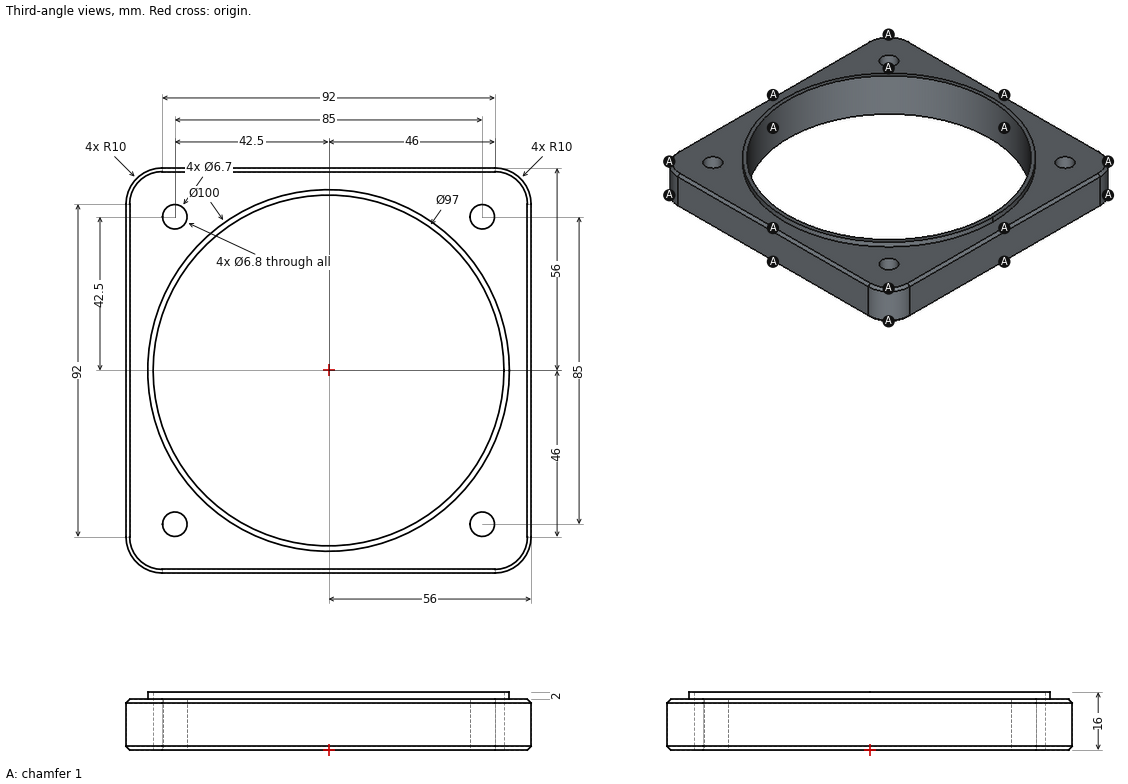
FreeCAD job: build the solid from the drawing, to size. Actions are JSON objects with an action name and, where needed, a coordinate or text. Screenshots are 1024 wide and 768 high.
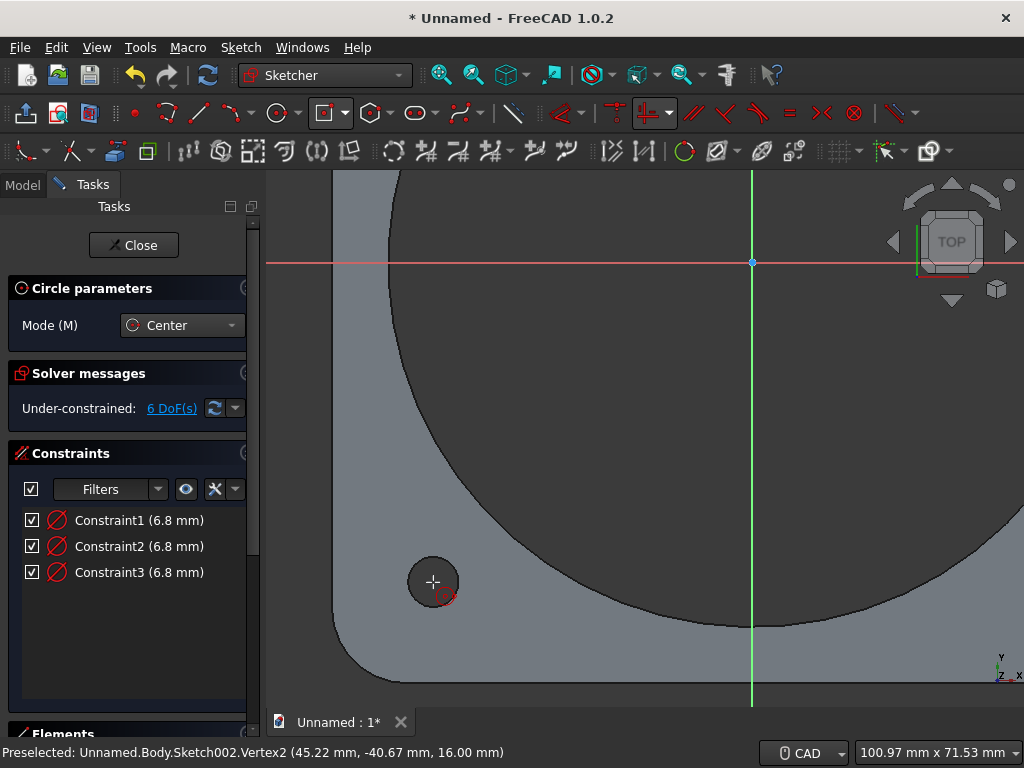
{"action": "left_click", "coordinate": [433, 582]}
{"action": "mouse_move", "coordinate": [451, 564]}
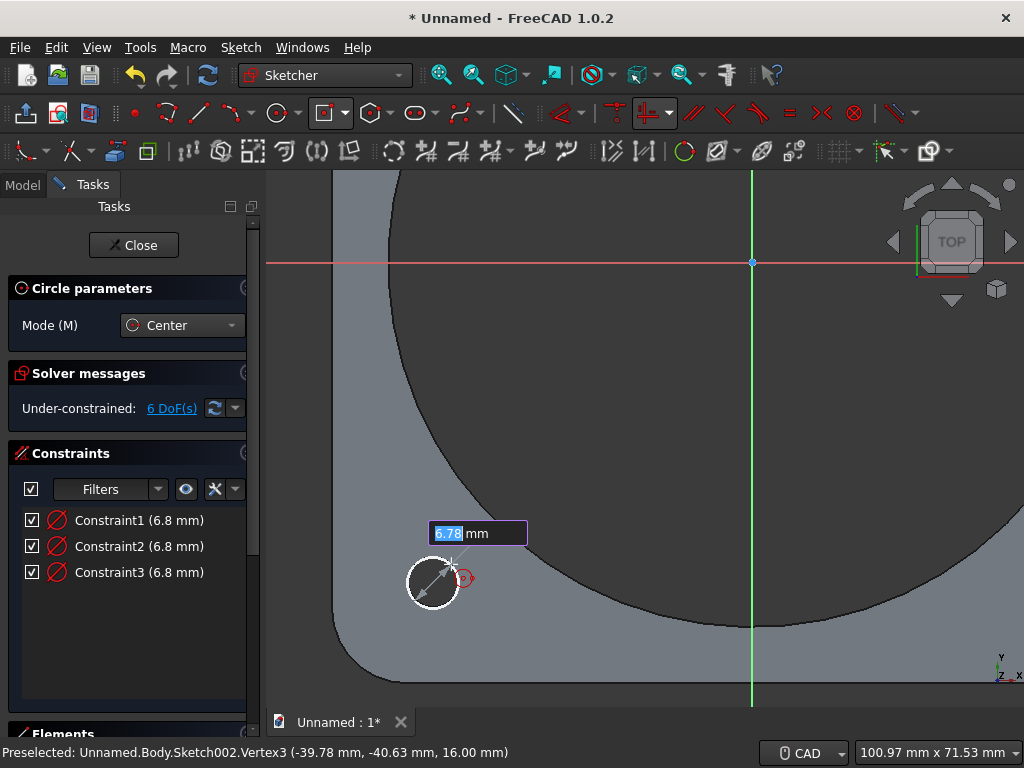
{"action": "type", "text": "6.8"}
{"action": "key", "text": "Return"}
{"action": "key", "text": "Escape"}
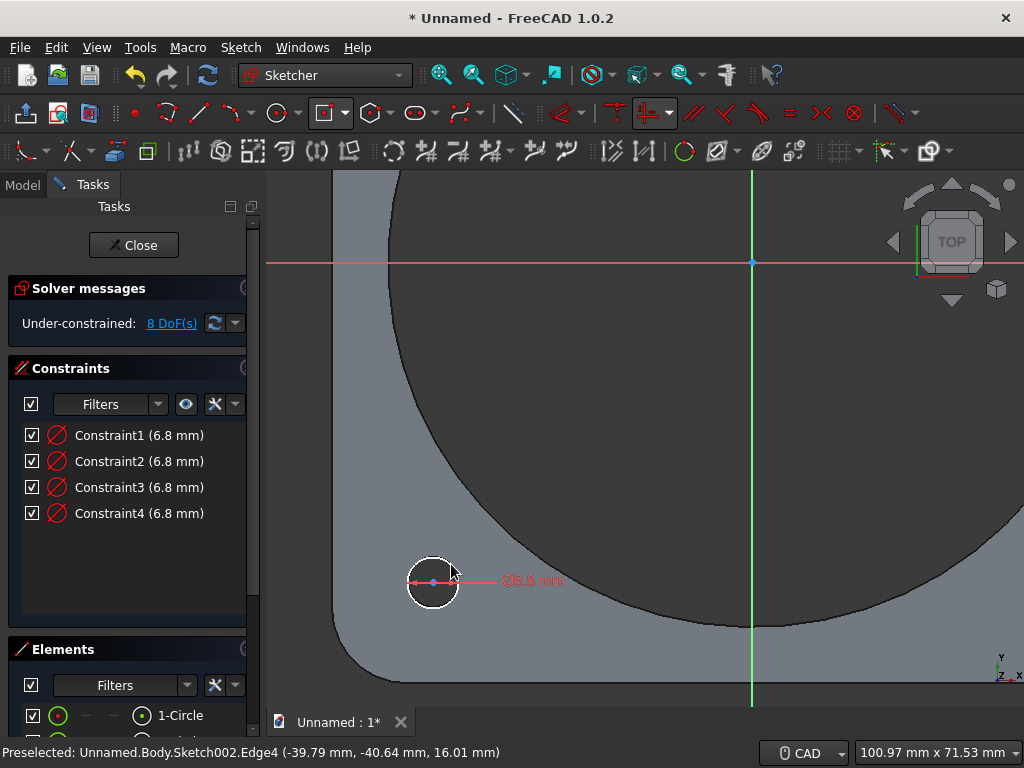
{"action": "scroll", "coordinate": [433, 582], "scroll_direction": "down", "scroll_amount": 4}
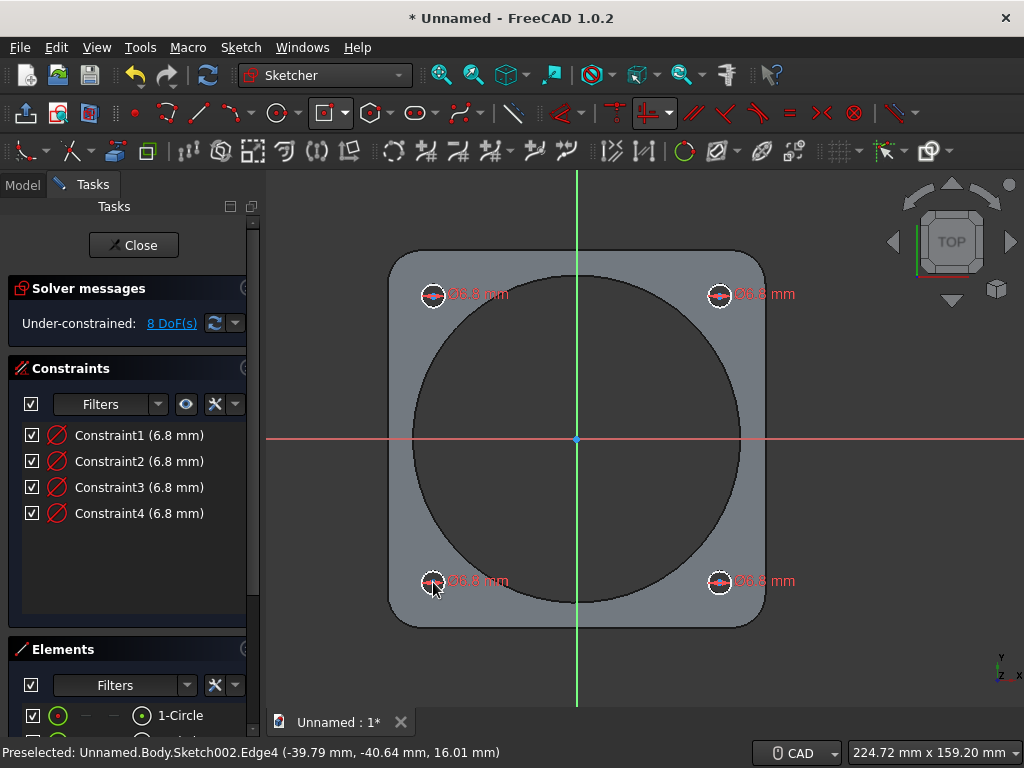
{"action": "left_click", "coordinate": [433, 296]}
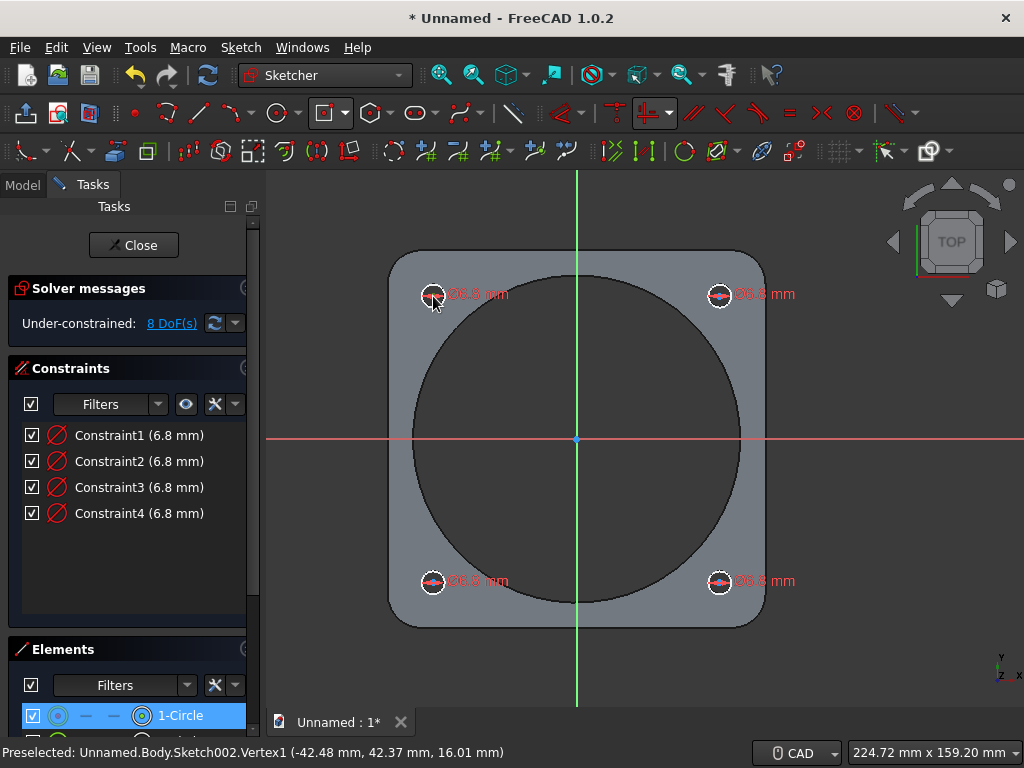
{"action": "left_click", "coordinate": [720, 296]}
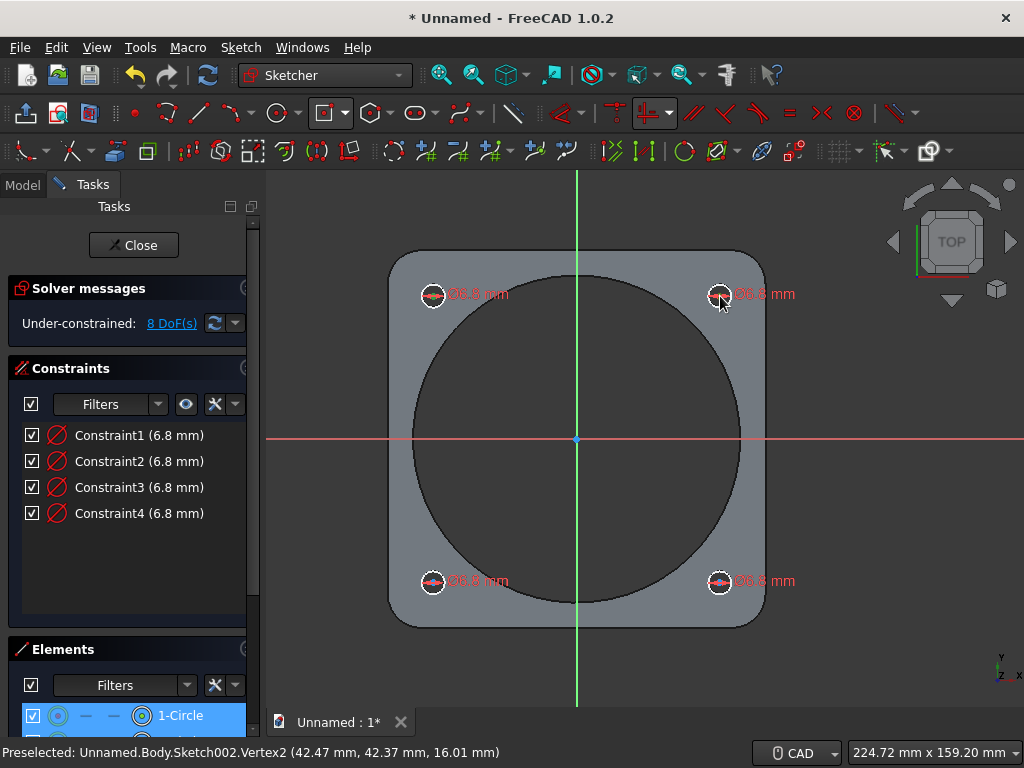
{"action": "left_click", "coordinate": [672, 114]}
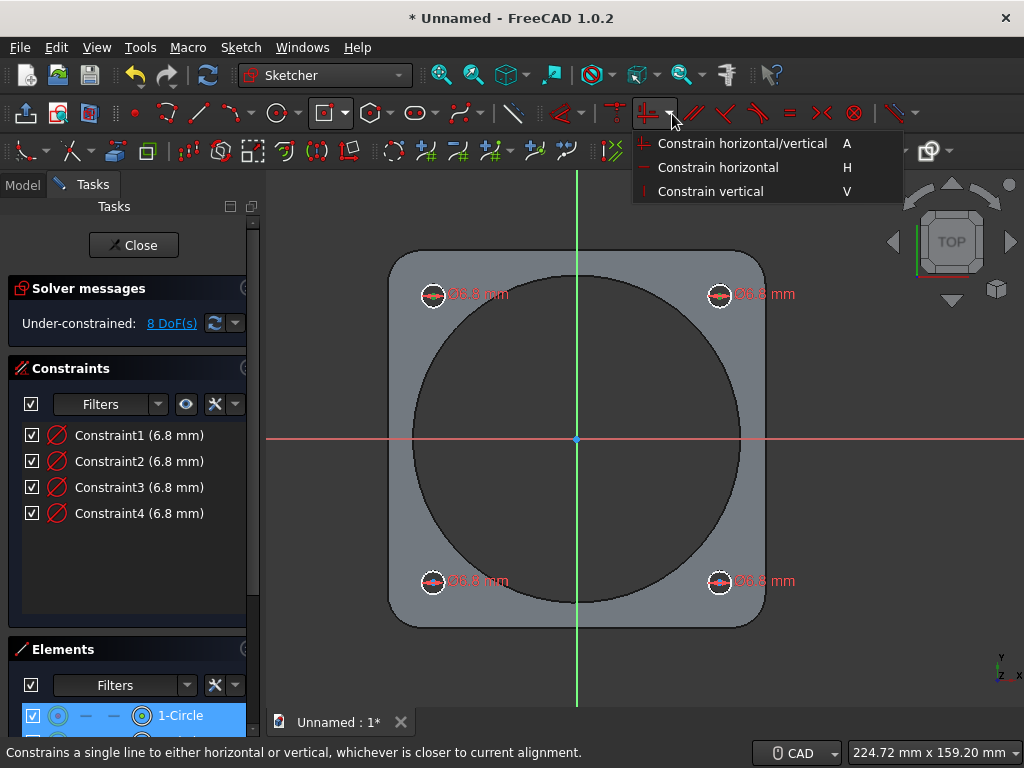
{"action": "left_click", "coordinate": [768, 167]}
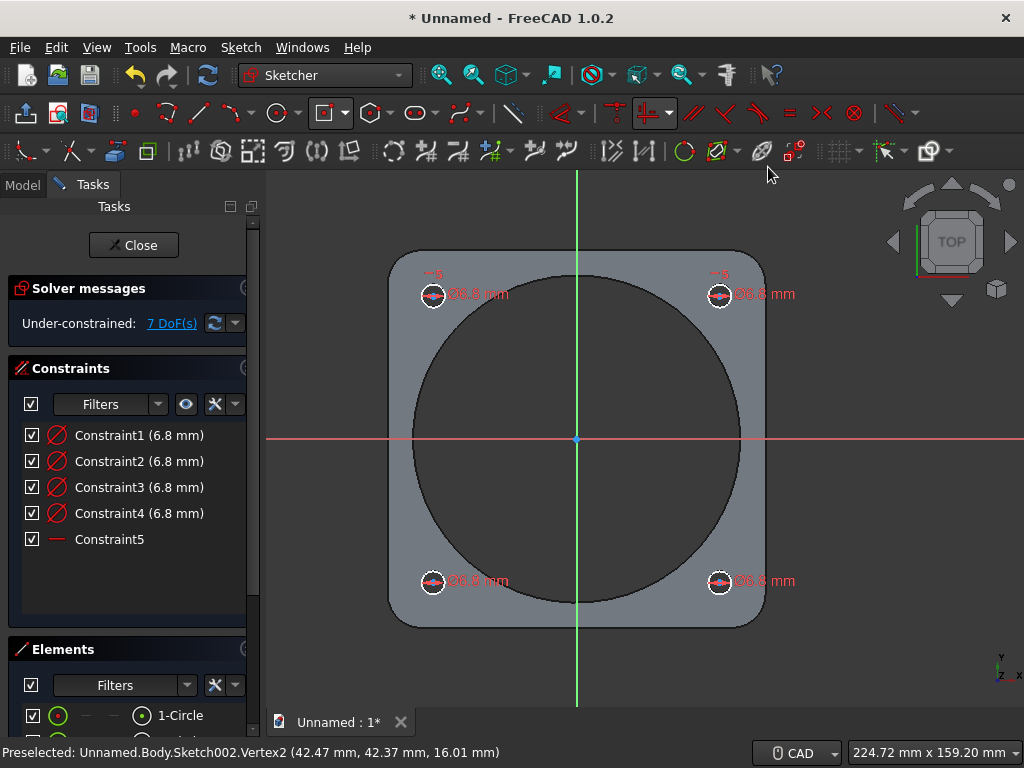
{"action": "left_click", "coordinate": [720, 296]}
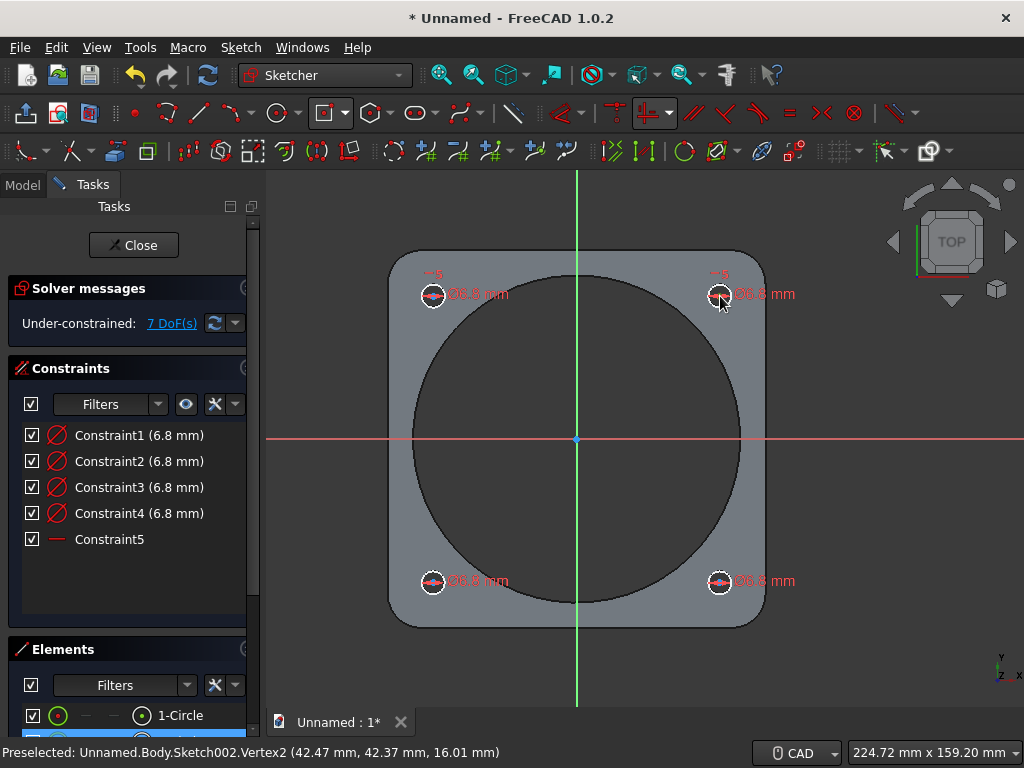
{"action": "left_click", "coordinate": [720, 583]}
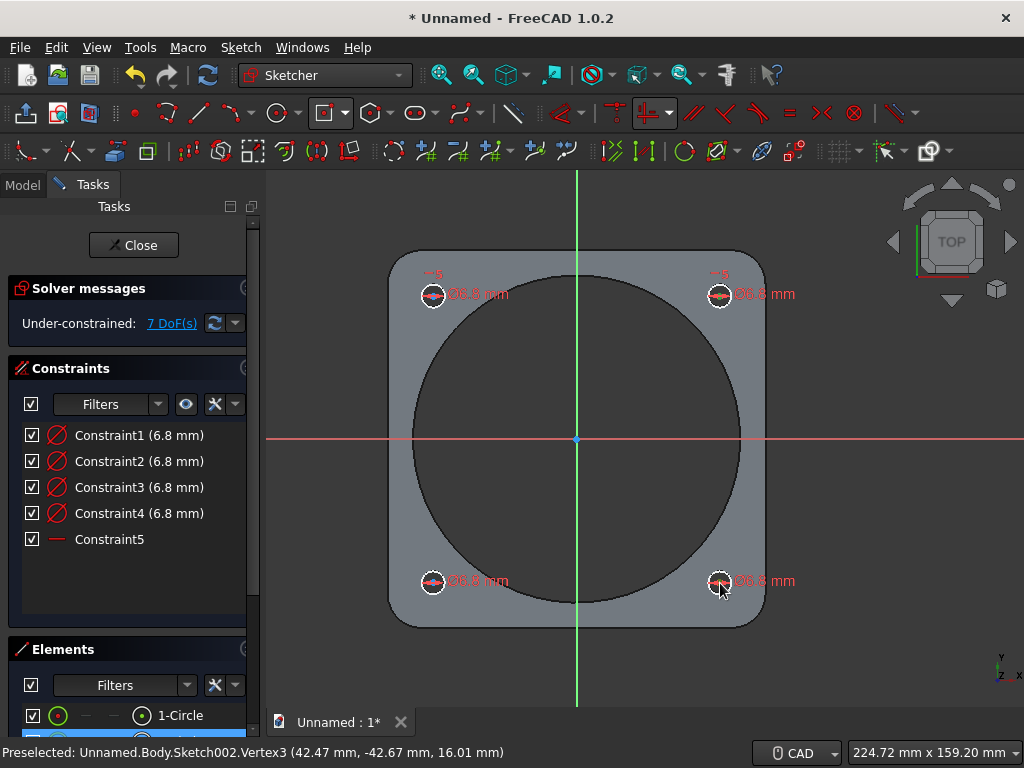
{"action": "left_click", "coordinate": [672, 114]}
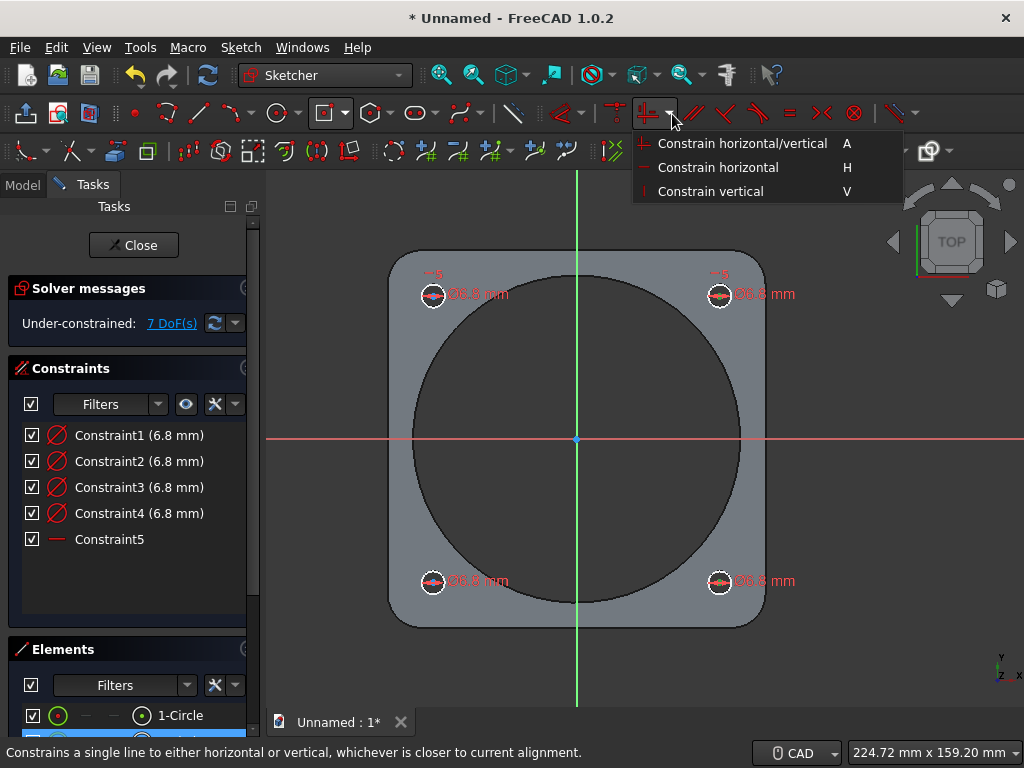
{"action": "left_click", "coordinate": [768, 191]}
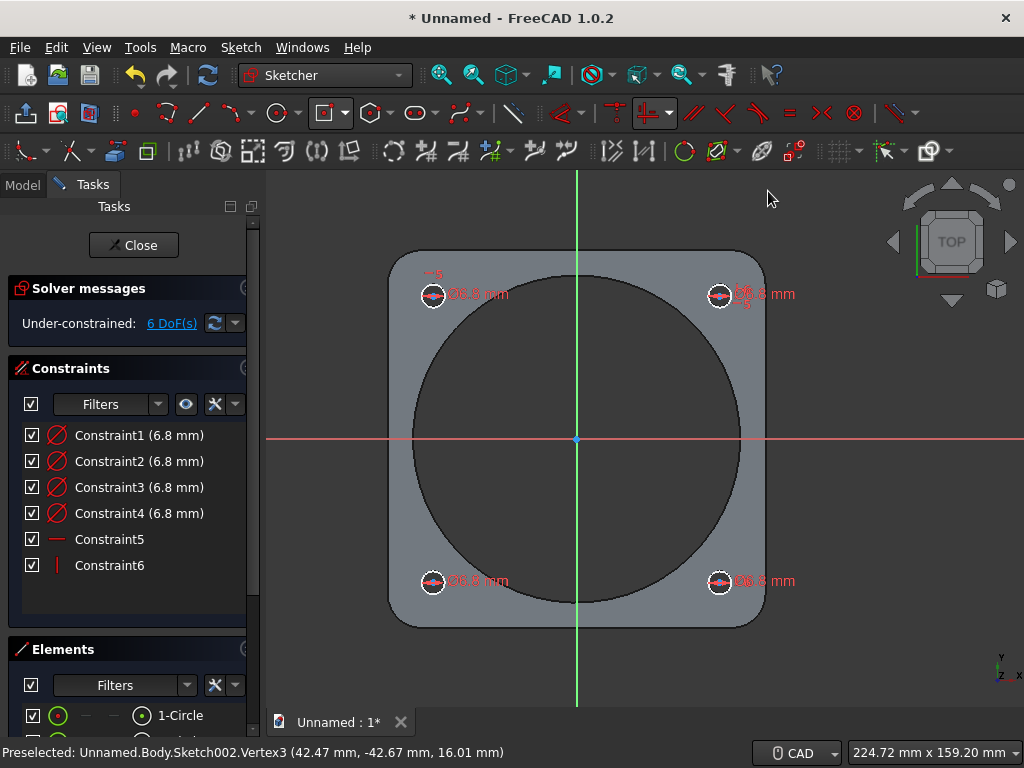
{"action": "left_click", "coordinate": [433, 296]}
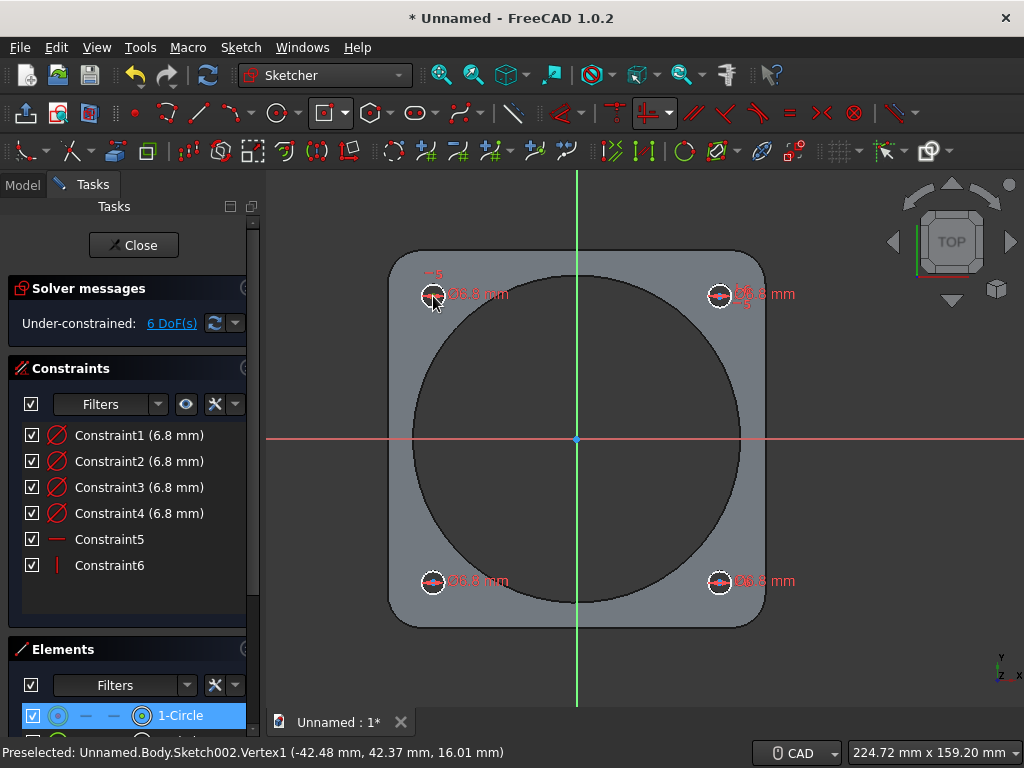
{"action": "left_click", "coordinate": [433, 583]}